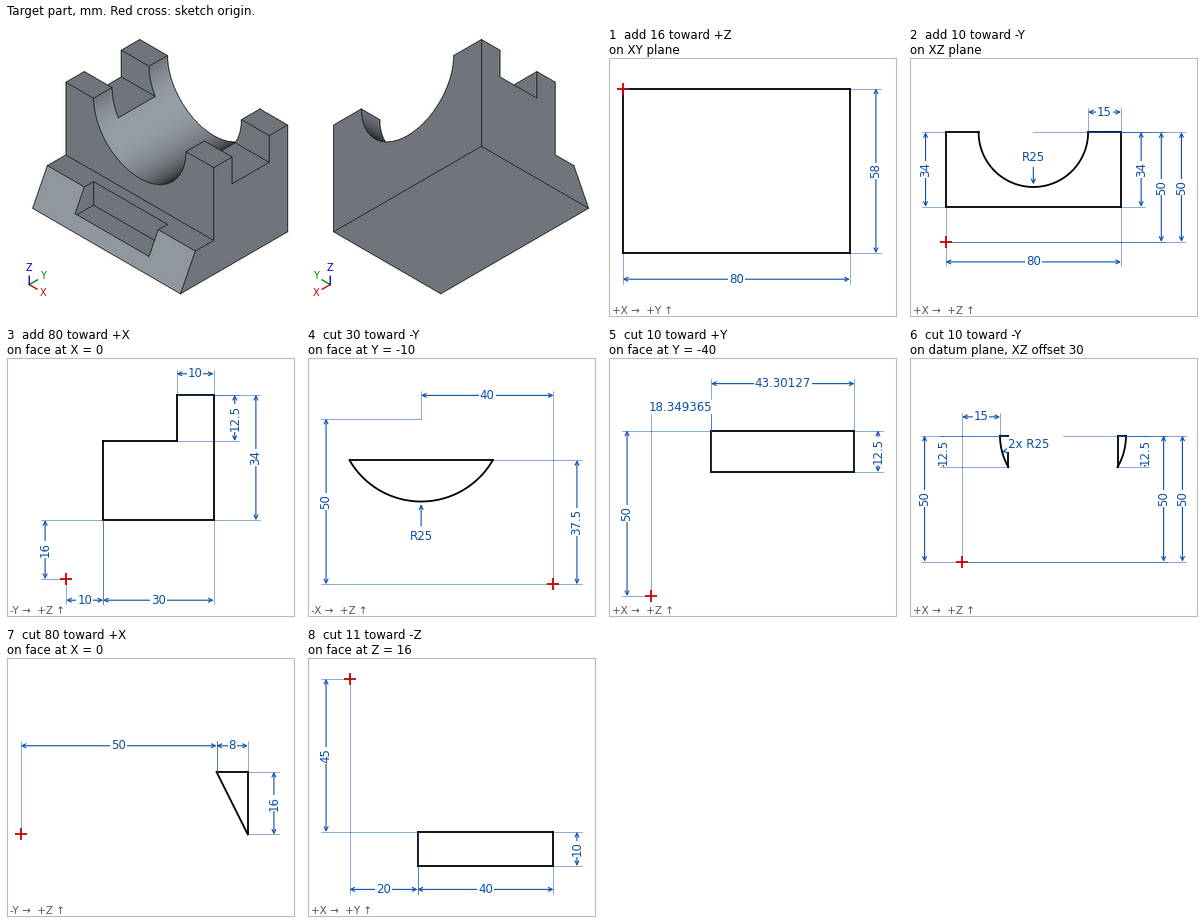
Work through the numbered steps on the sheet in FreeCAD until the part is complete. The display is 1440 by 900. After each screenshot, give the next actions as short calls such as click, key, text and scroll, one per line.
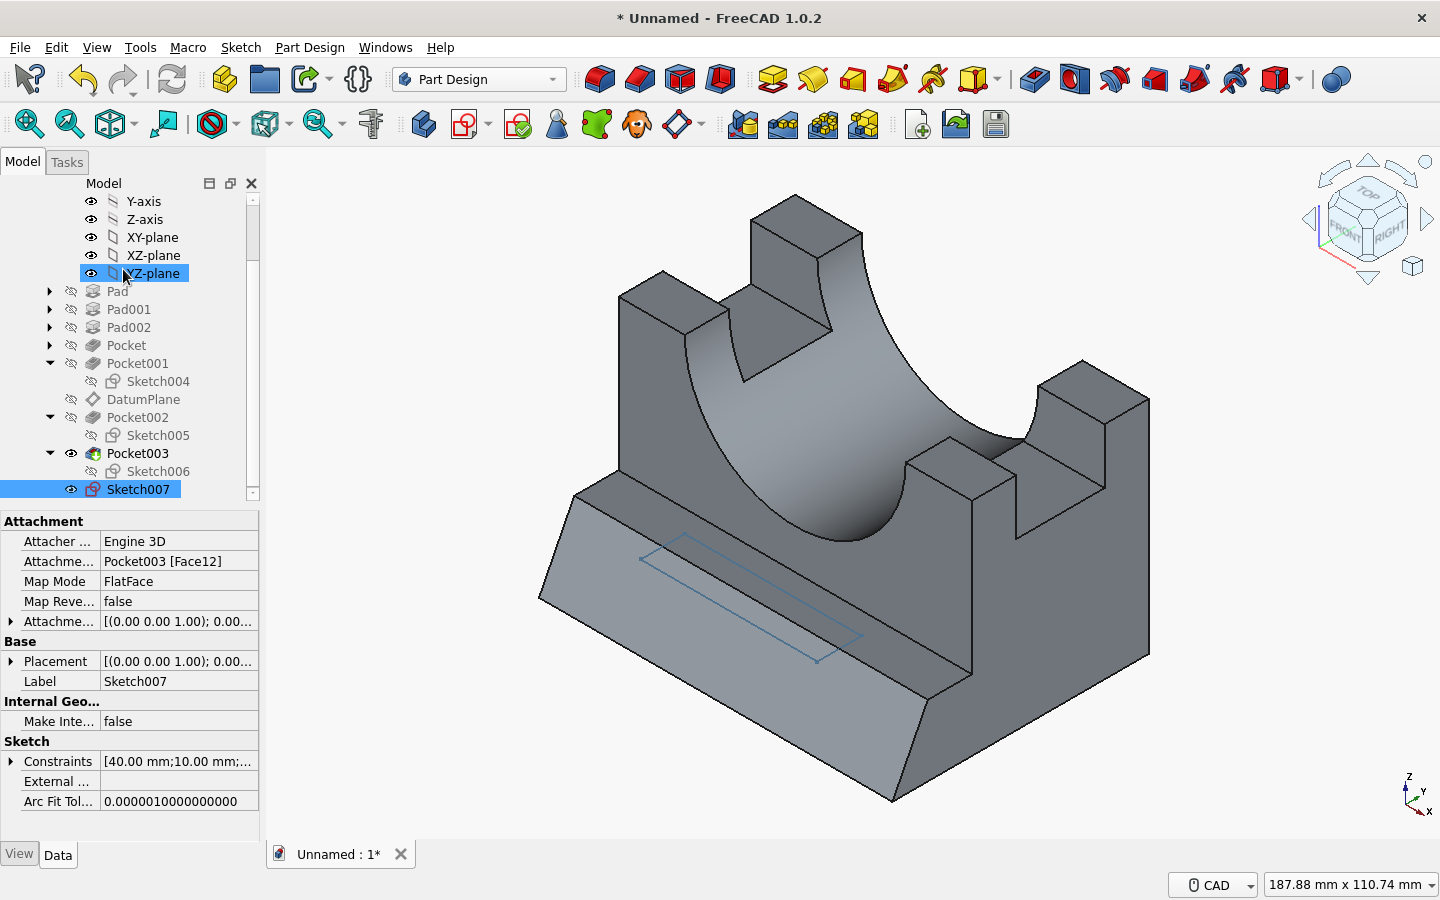
click(1036, 80)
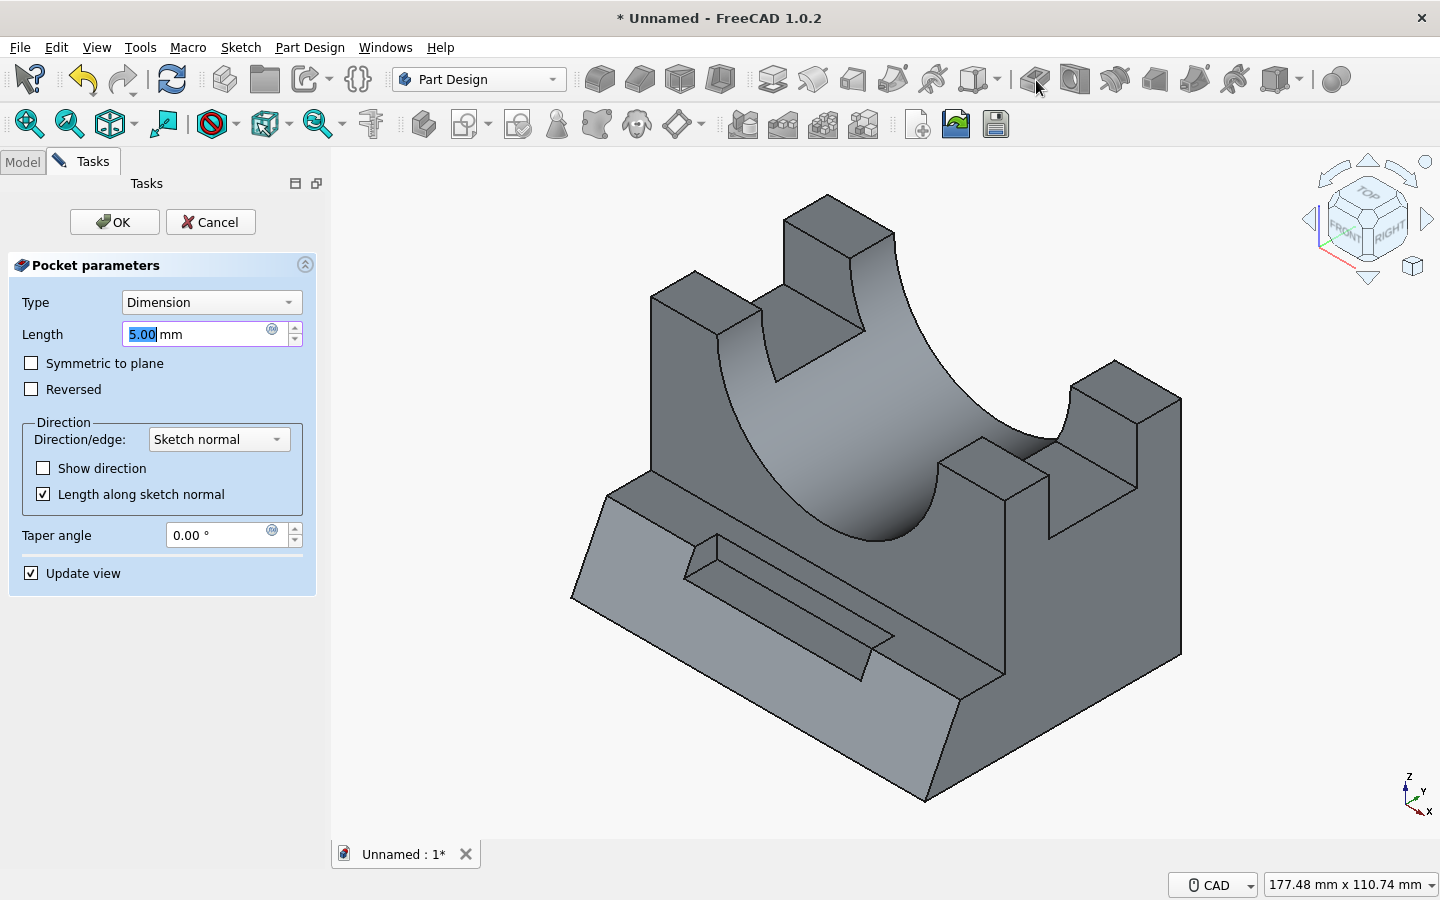
text(11)
key(Tab)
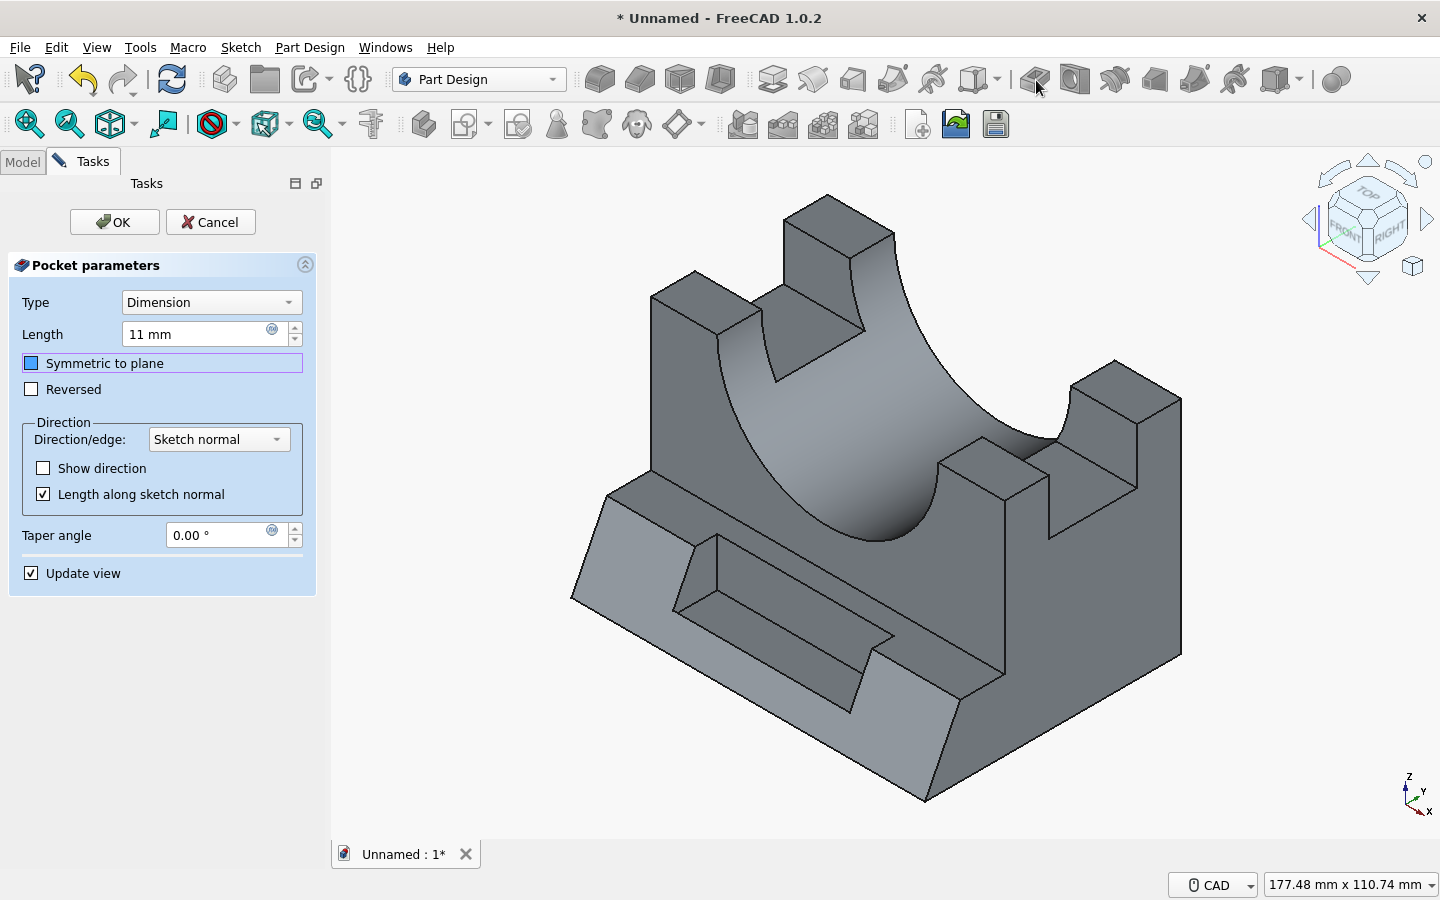
click(115, 222)